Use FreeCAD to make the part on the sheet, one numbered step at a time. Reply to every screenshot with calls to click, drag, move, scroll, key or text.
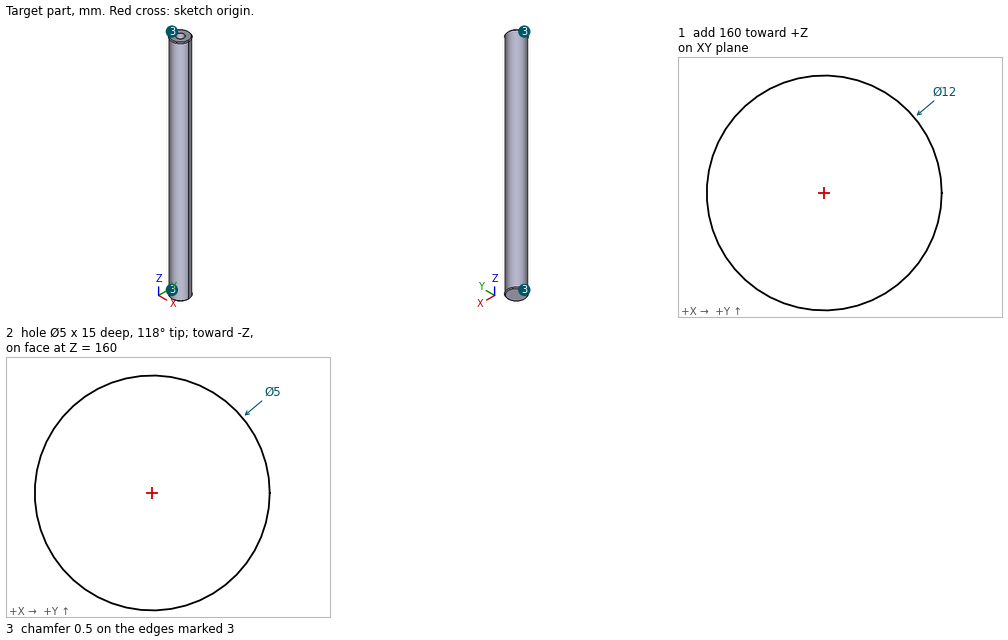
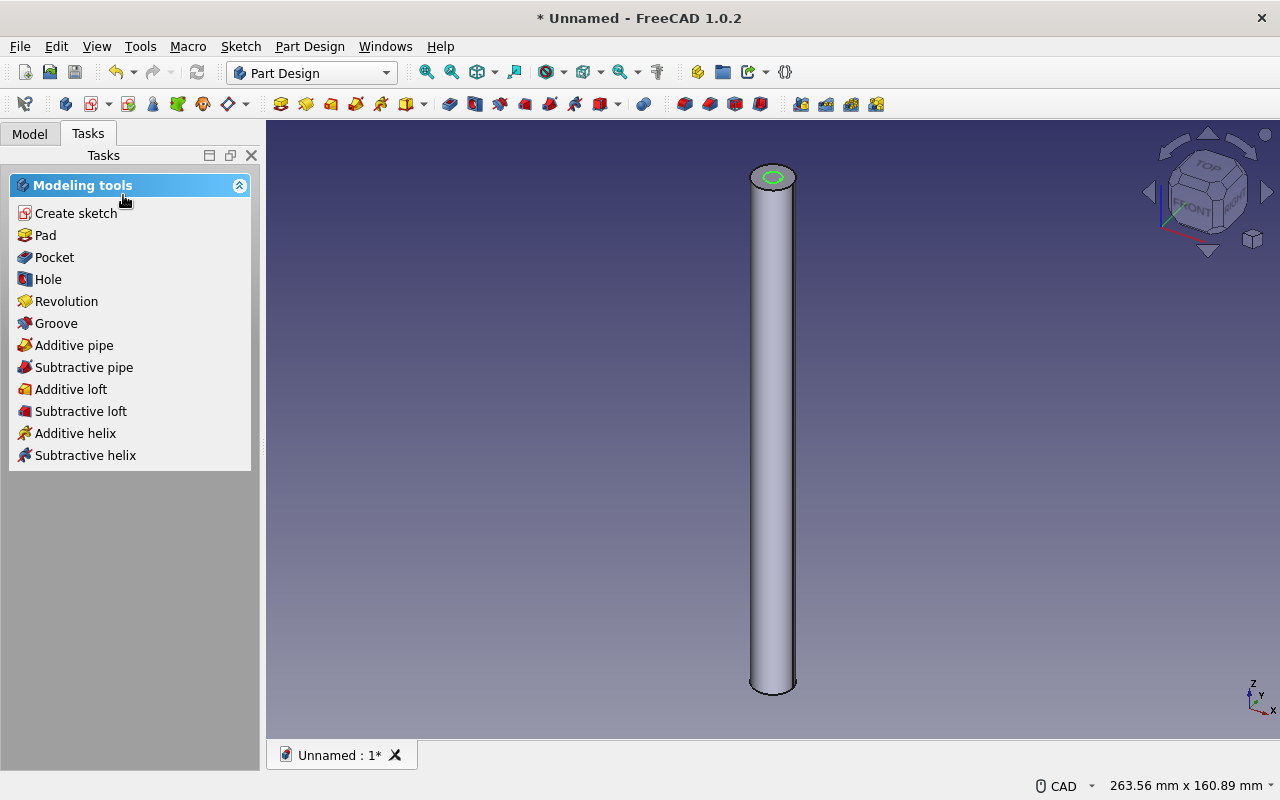
click(475, 104)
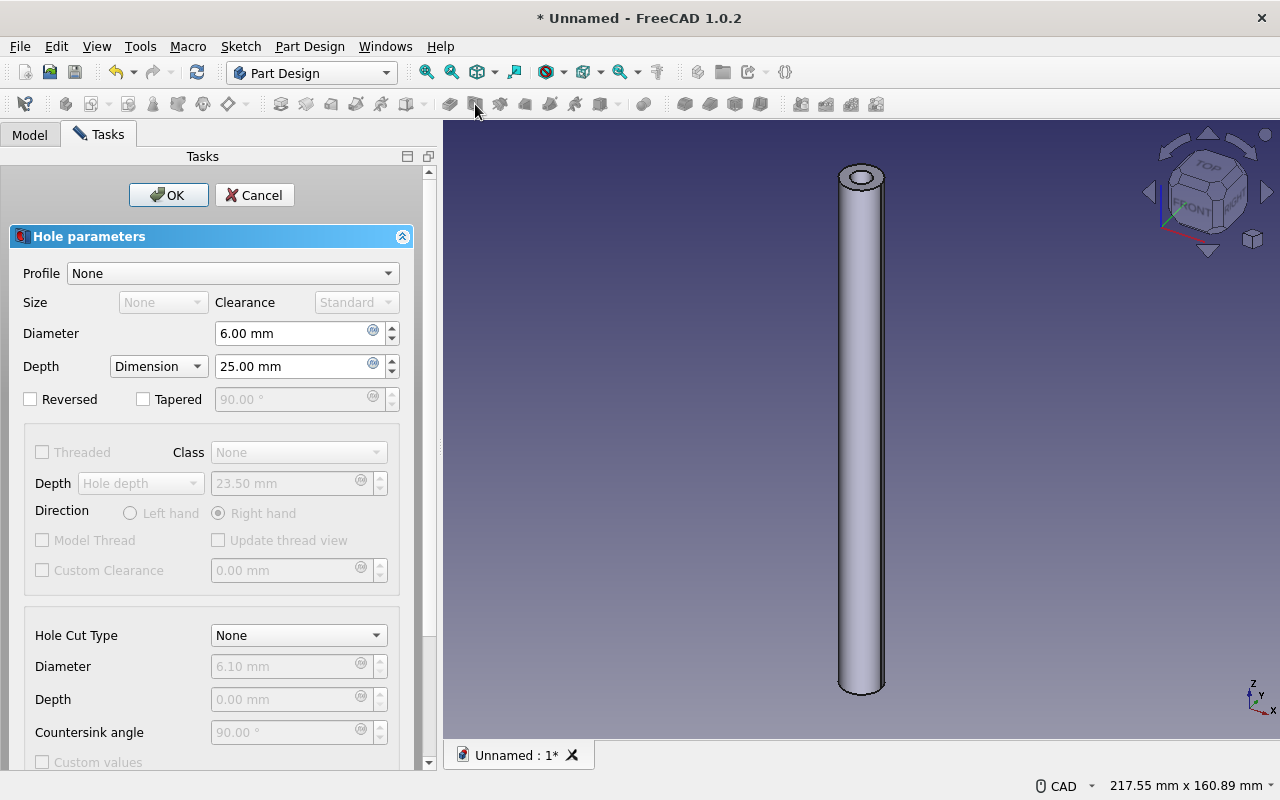
triple_click(300, 334)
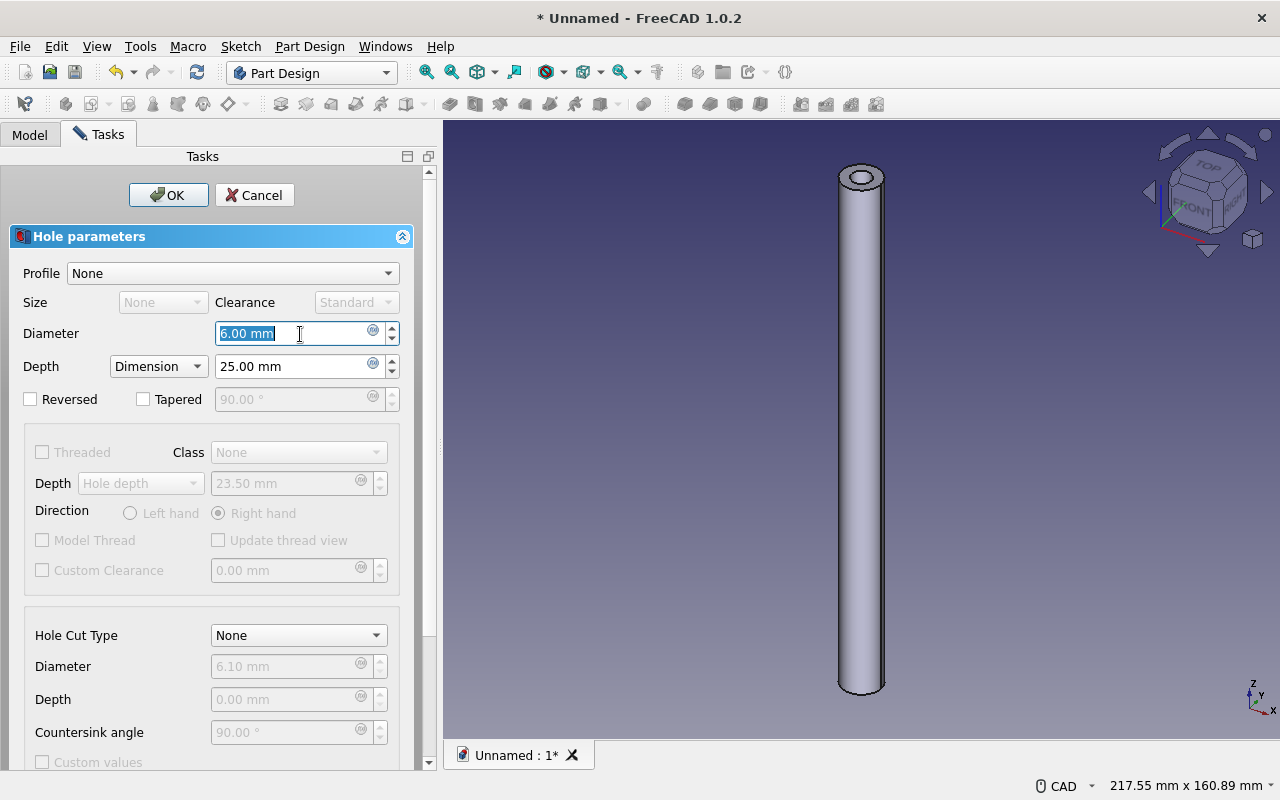
text(5)
key(Tab)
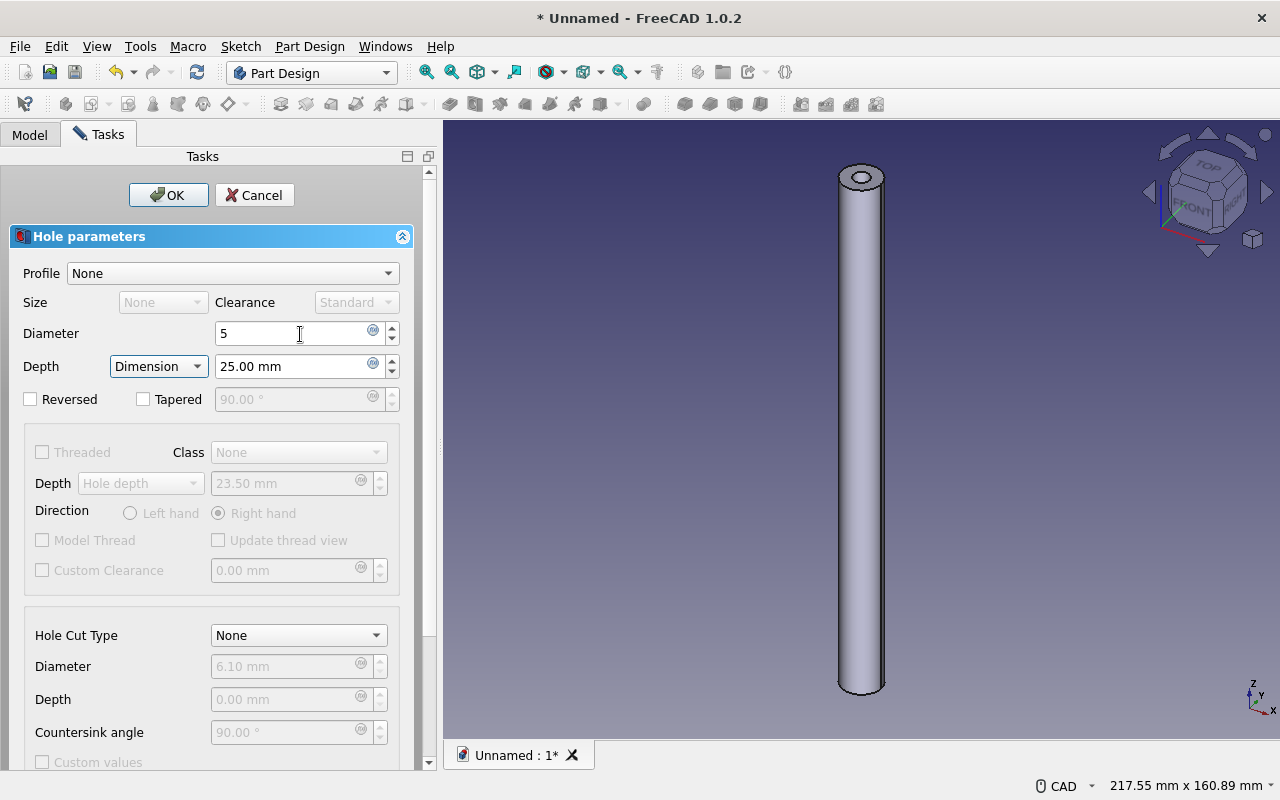
triple_click(300, 366)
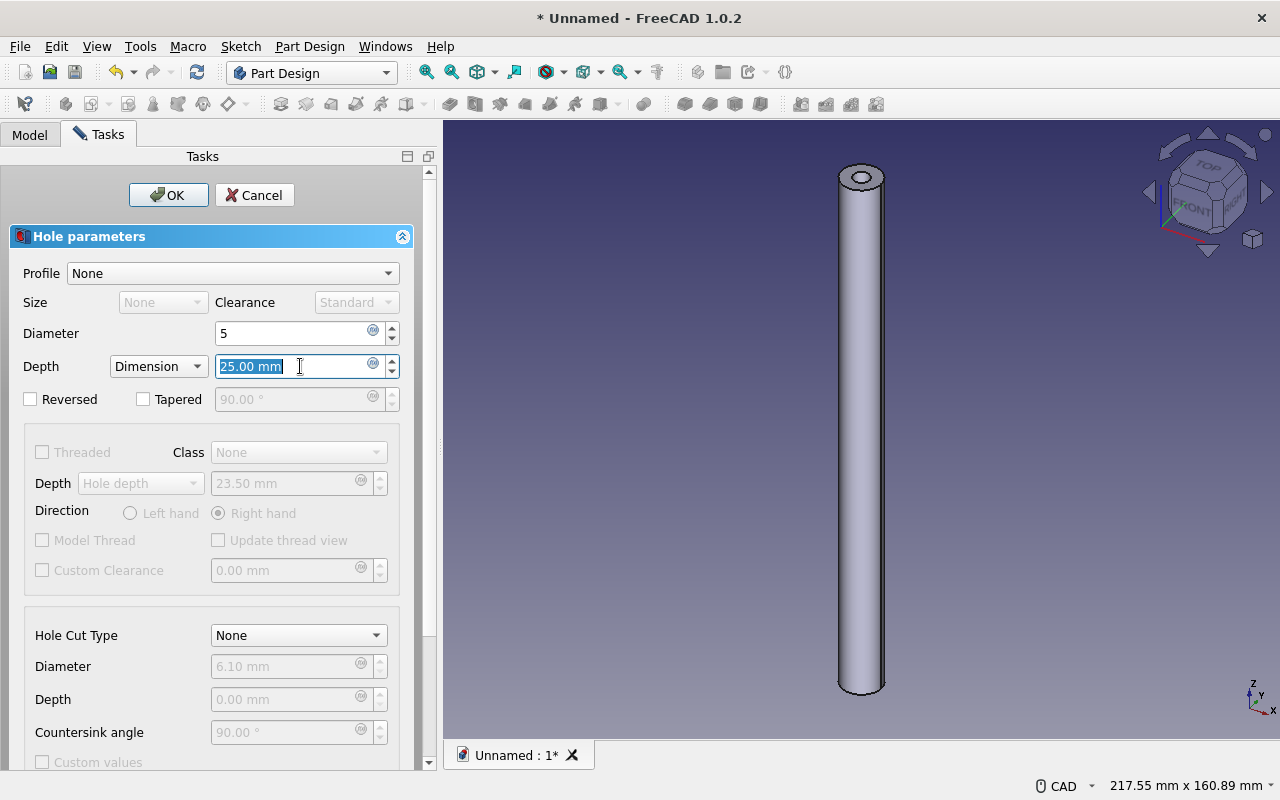
text(15)
key(Tab)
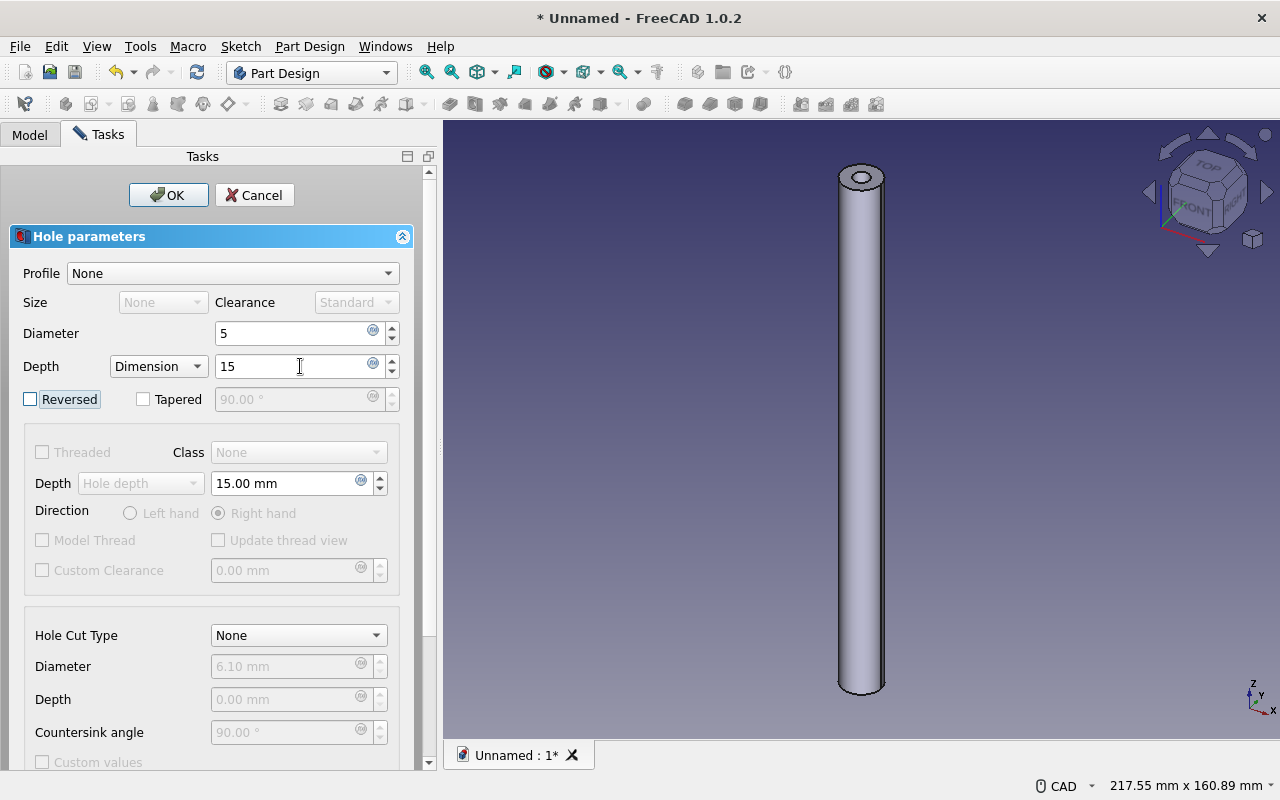
click(169, 195)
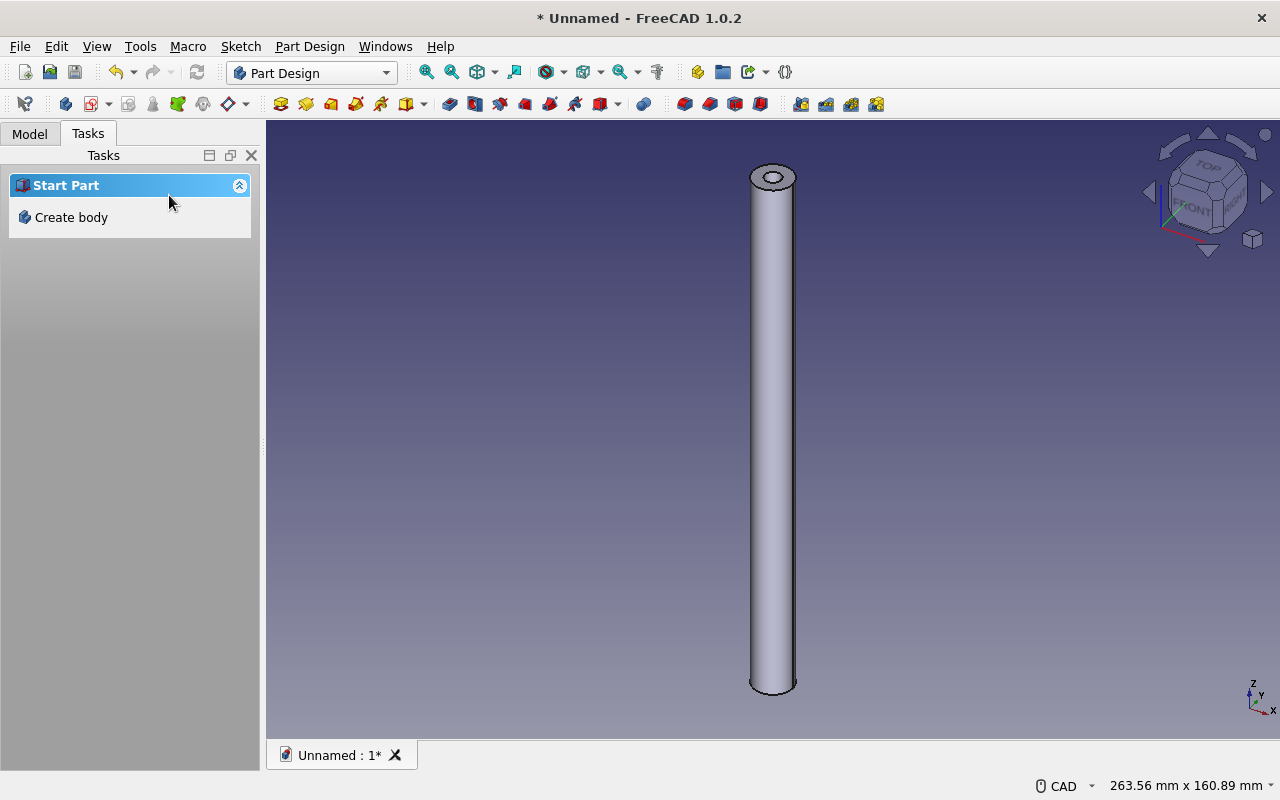
click(764, 164)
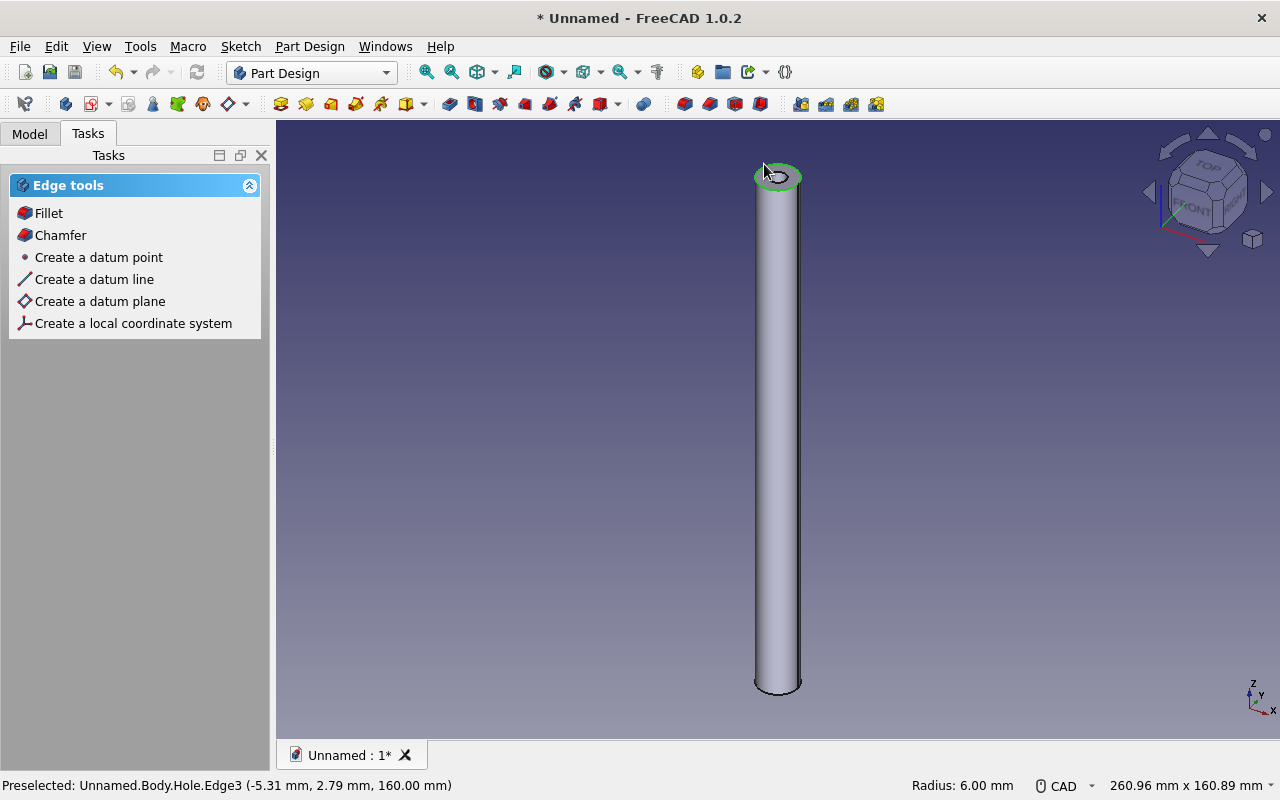
key(0)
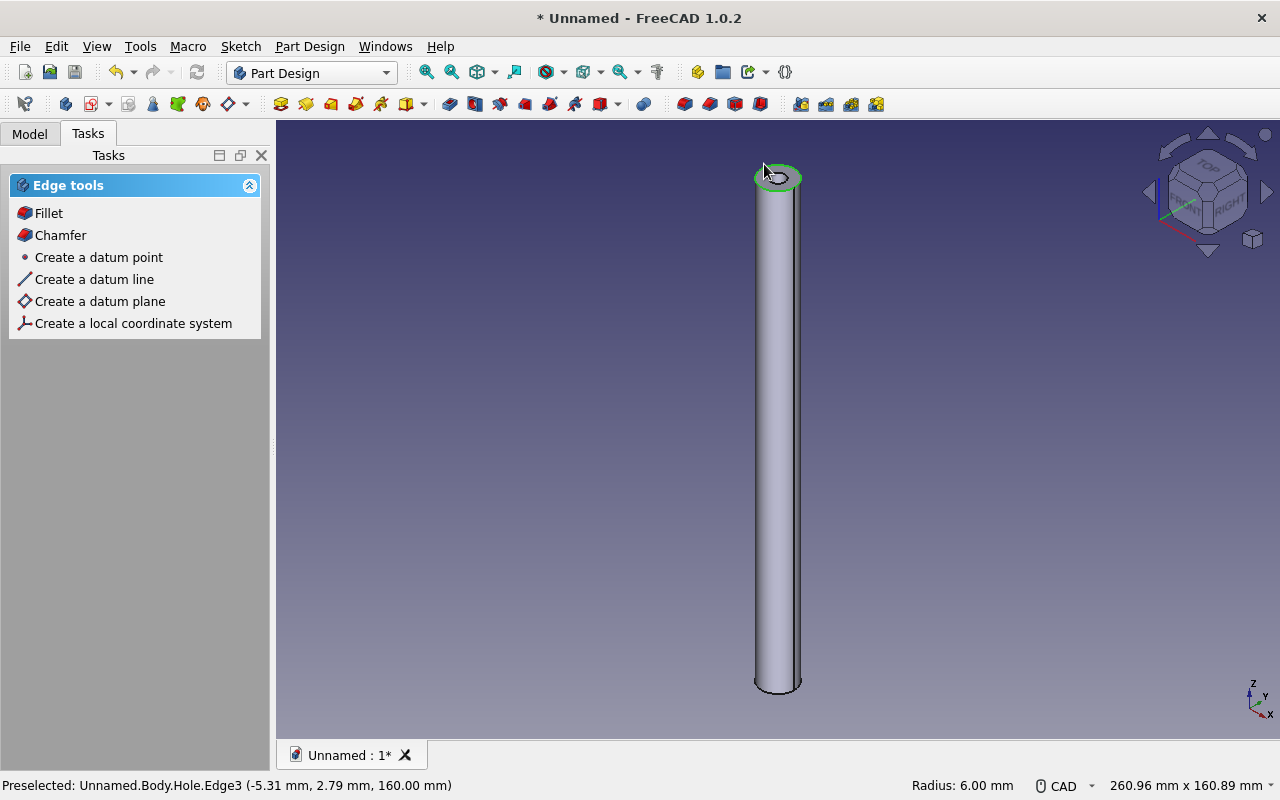
click(757, 686, ctrl)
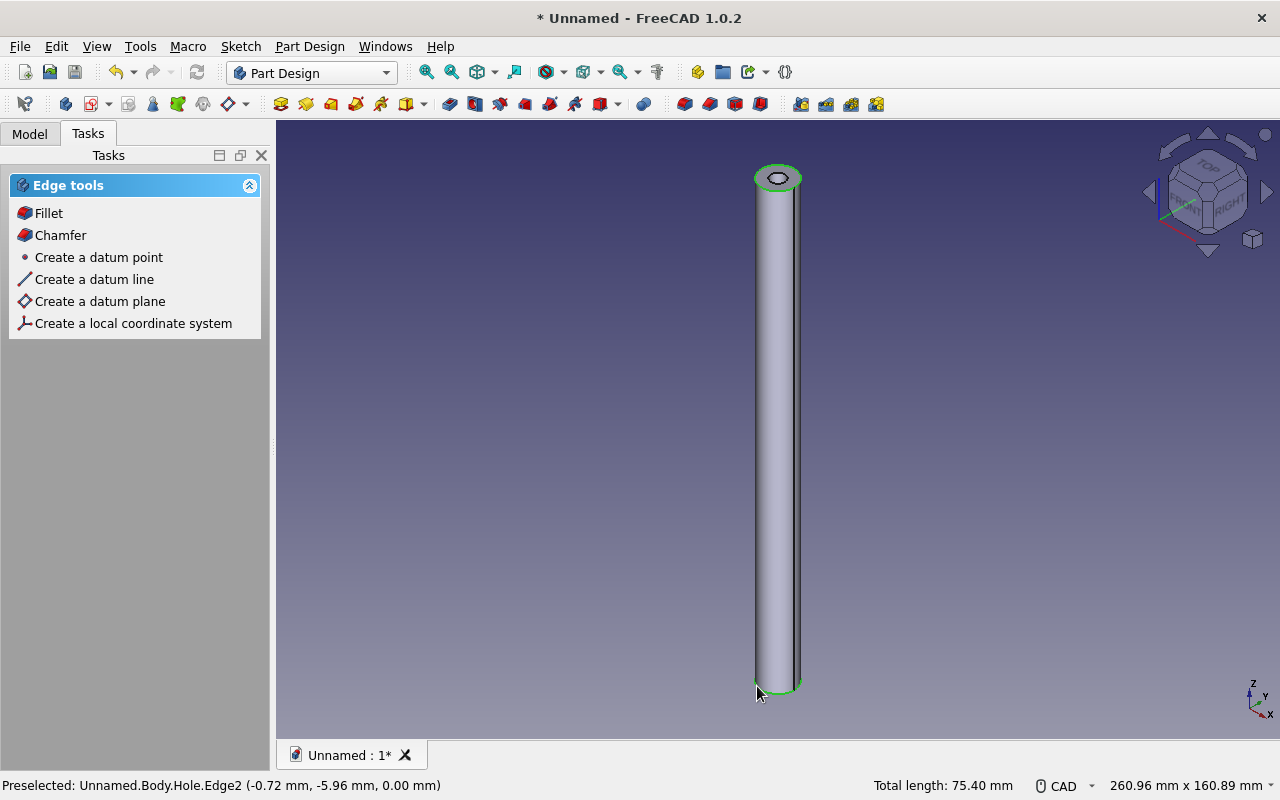
click(710, 104)